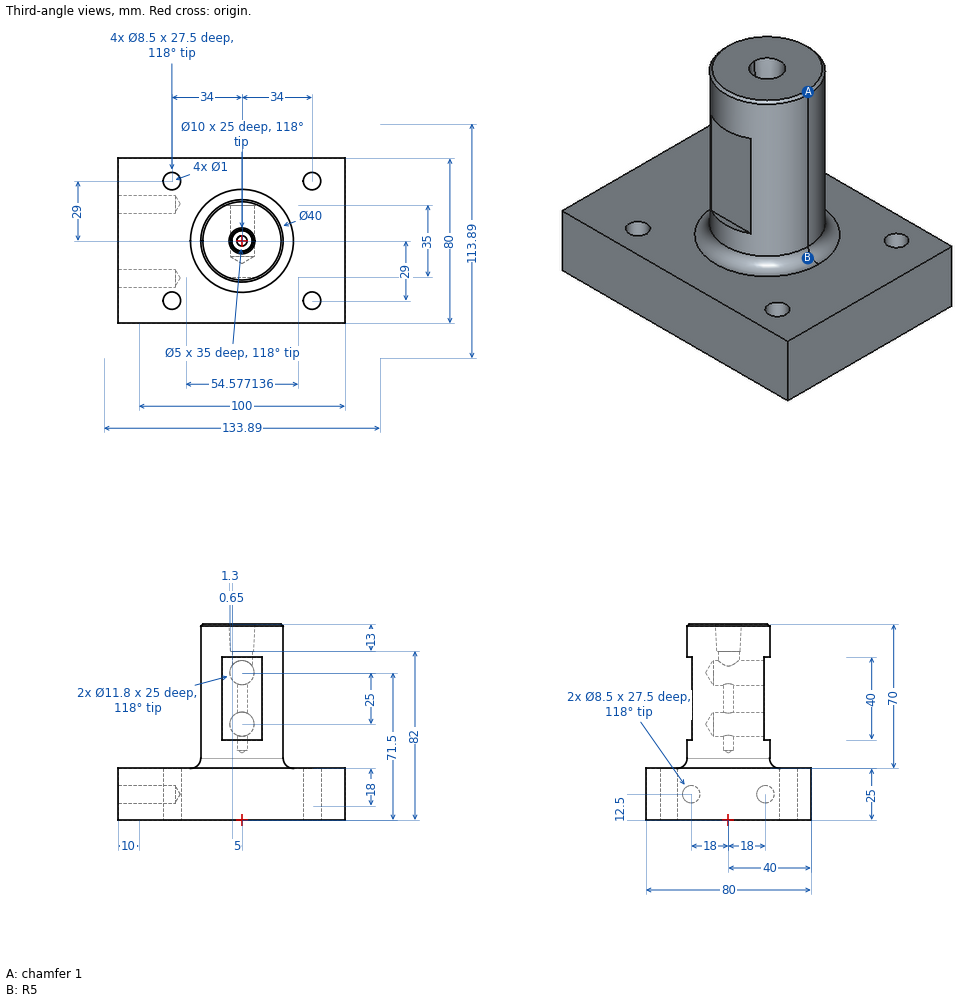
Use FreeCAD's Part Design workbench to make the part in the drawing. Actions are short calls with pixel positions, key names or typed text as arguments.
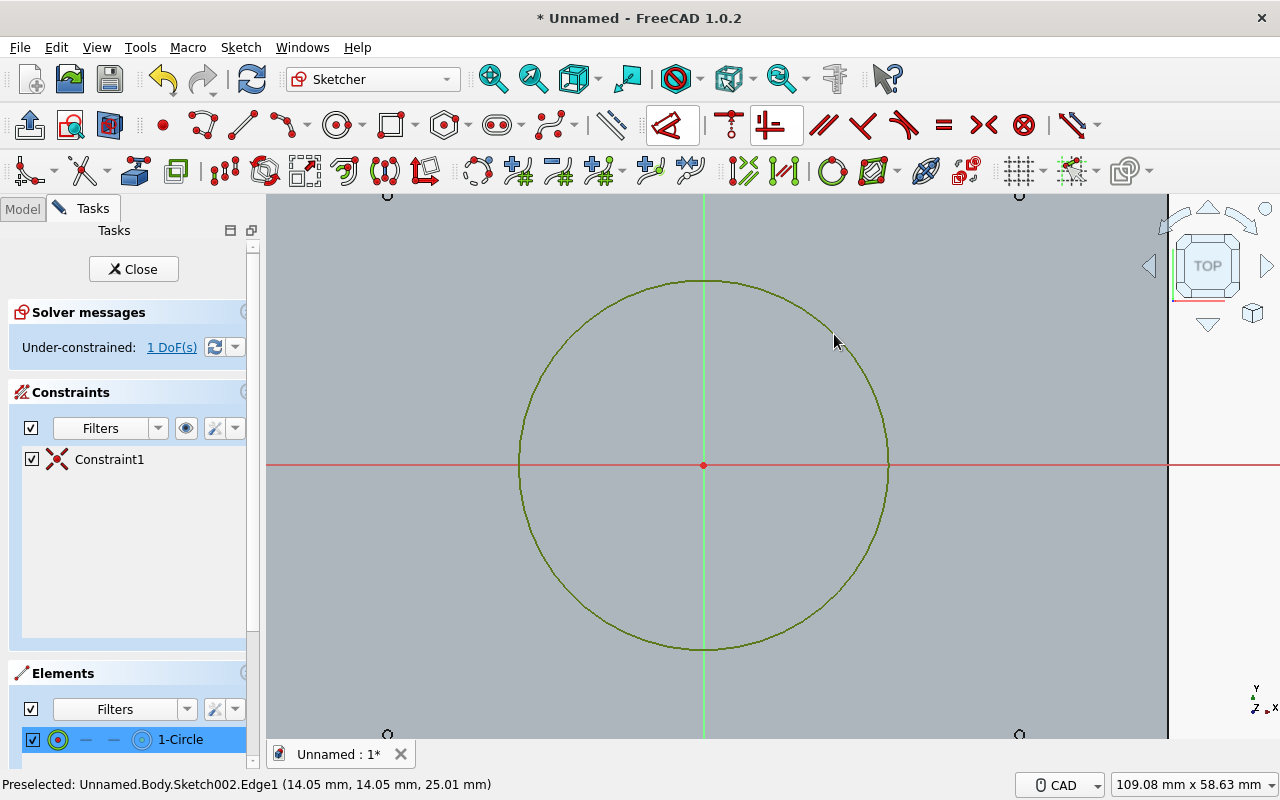
click(694, 126)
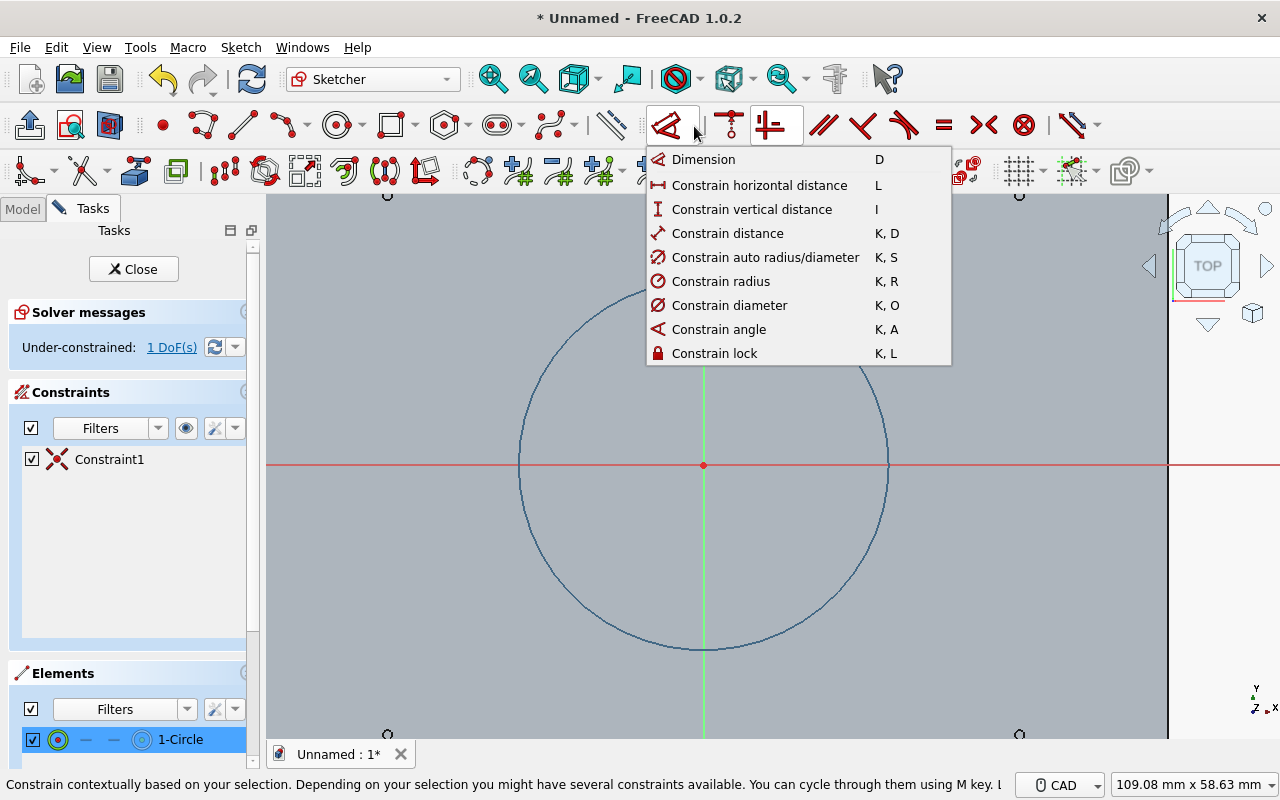
click(799, 305)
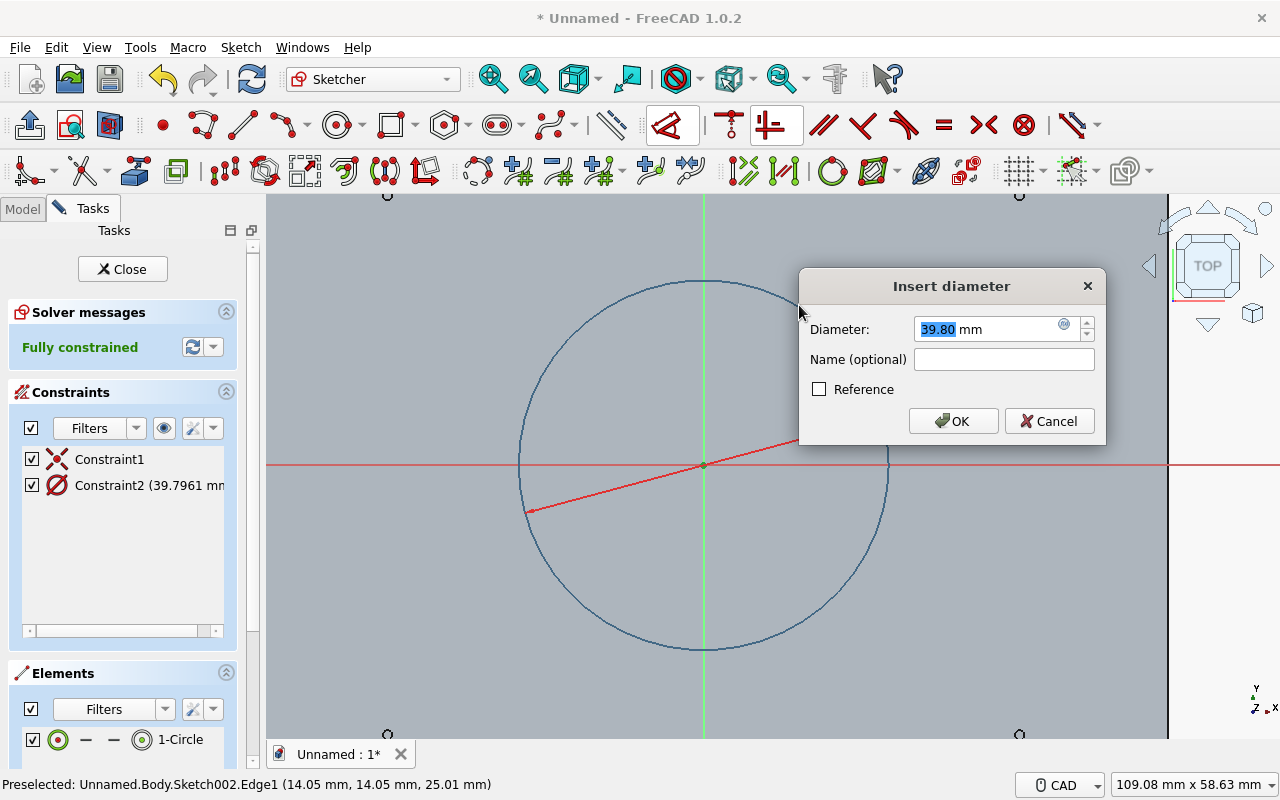
text(40)
key(Return)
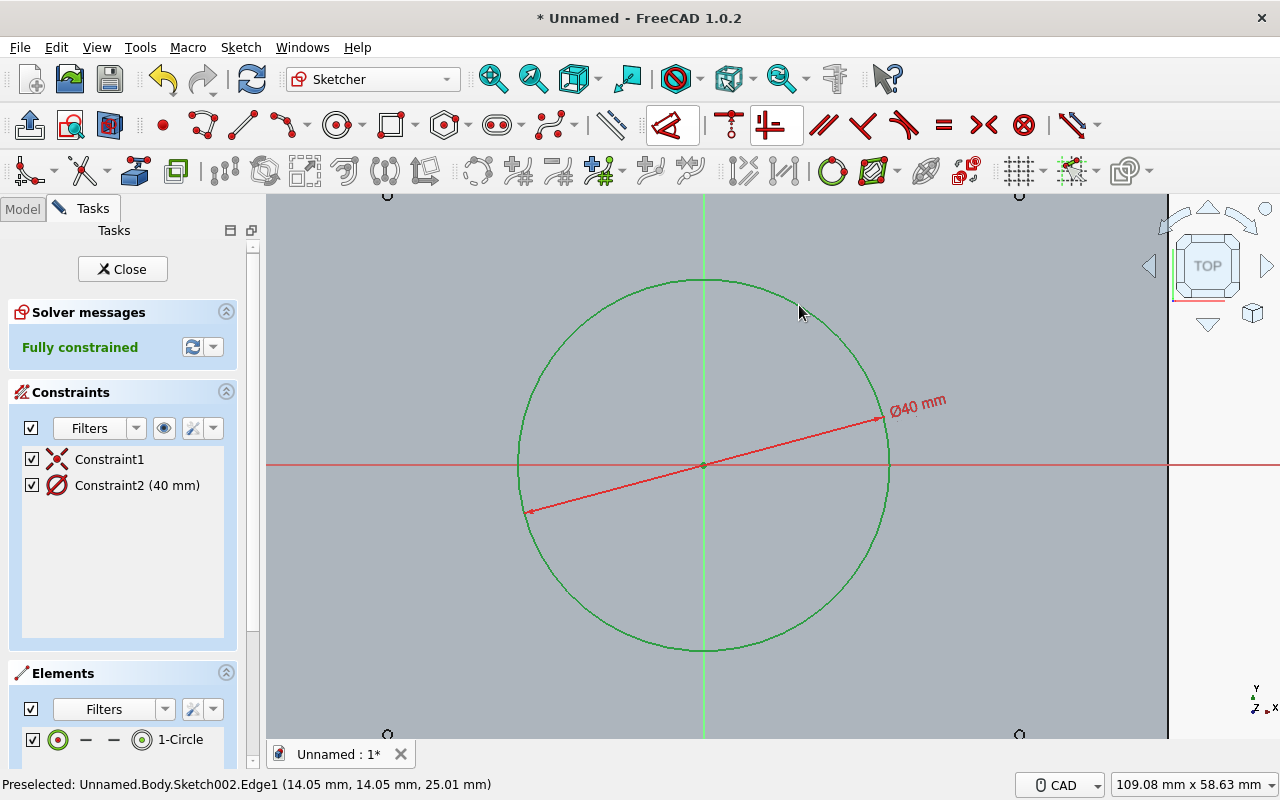
click(123, 269)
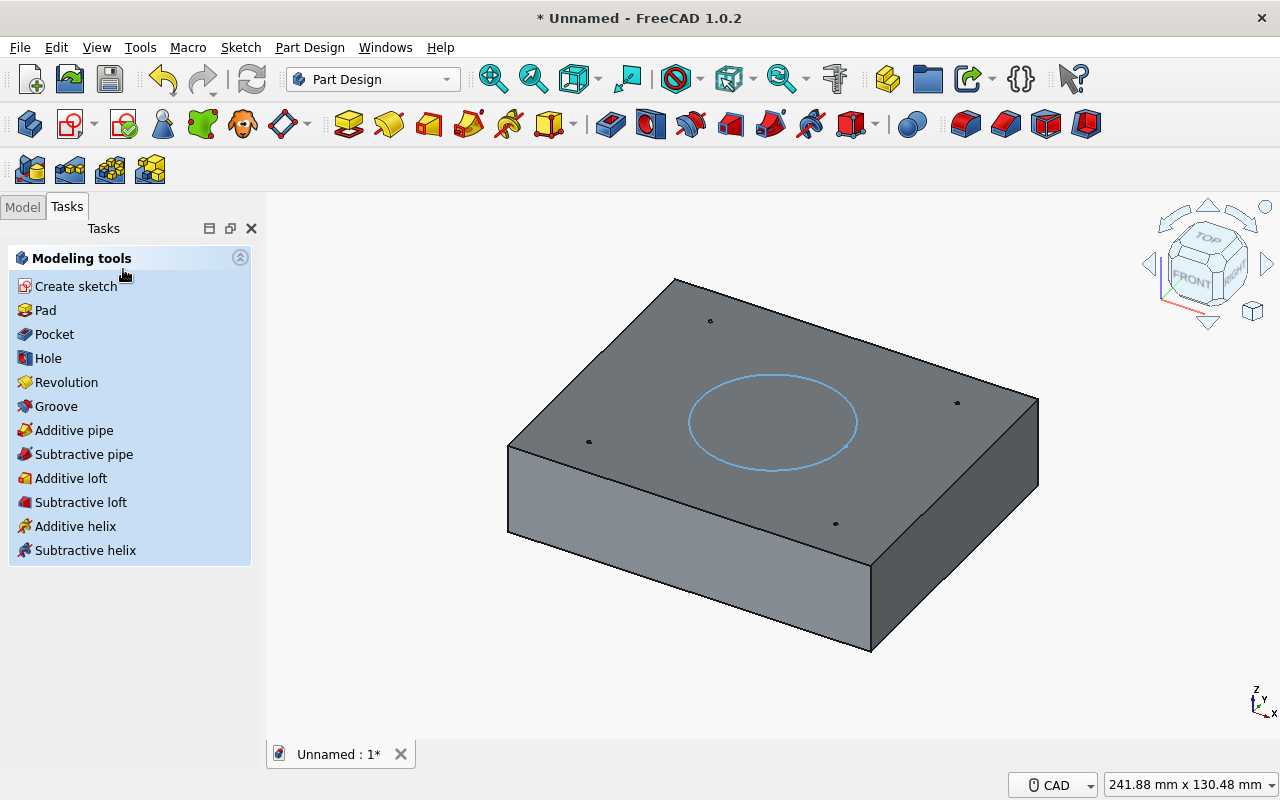
click(350, 124)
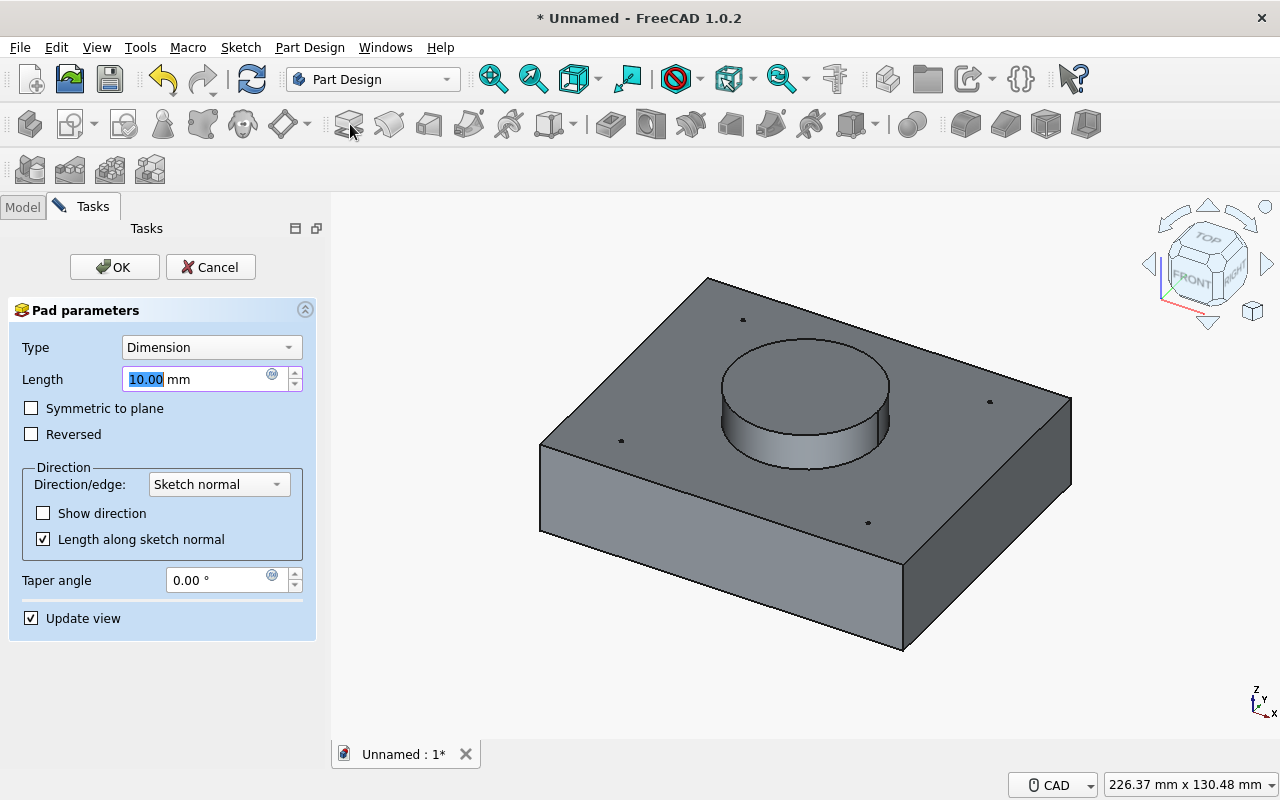
text(70)
key(Tab)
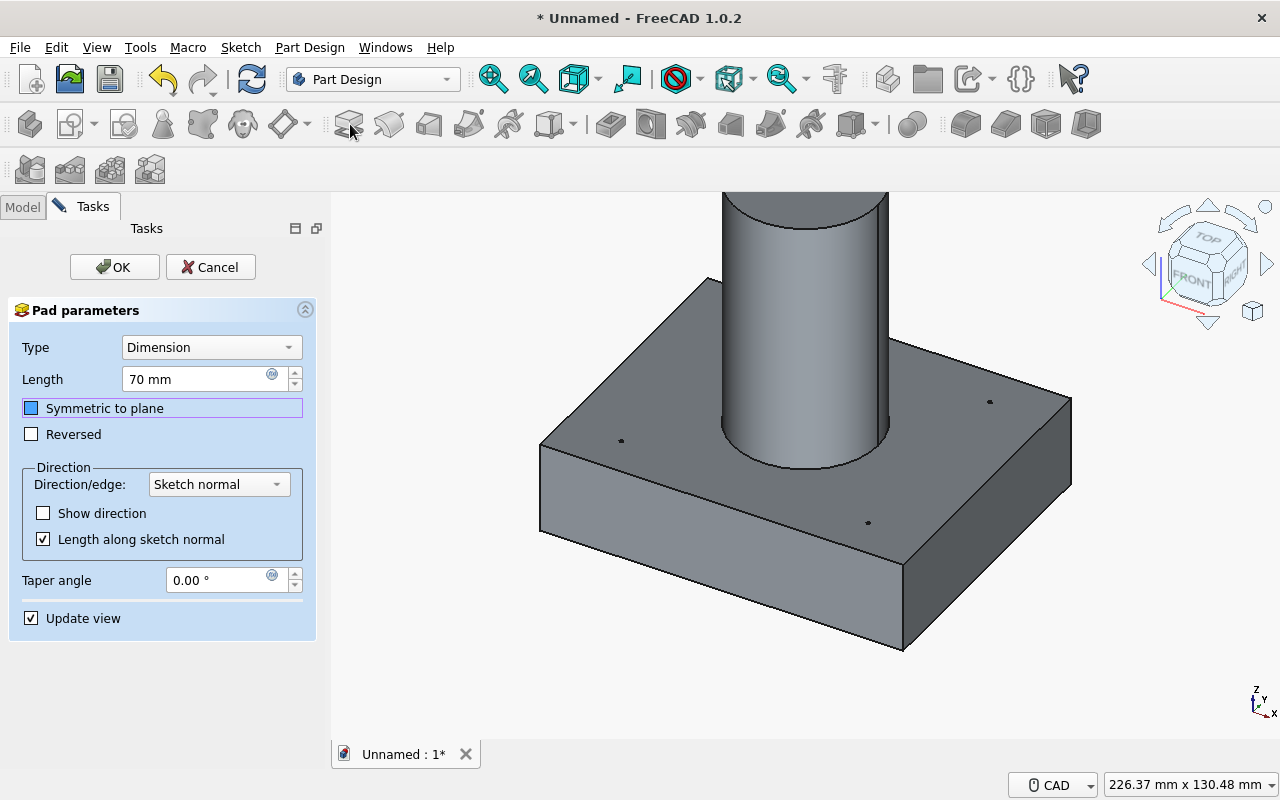
click(115, 267)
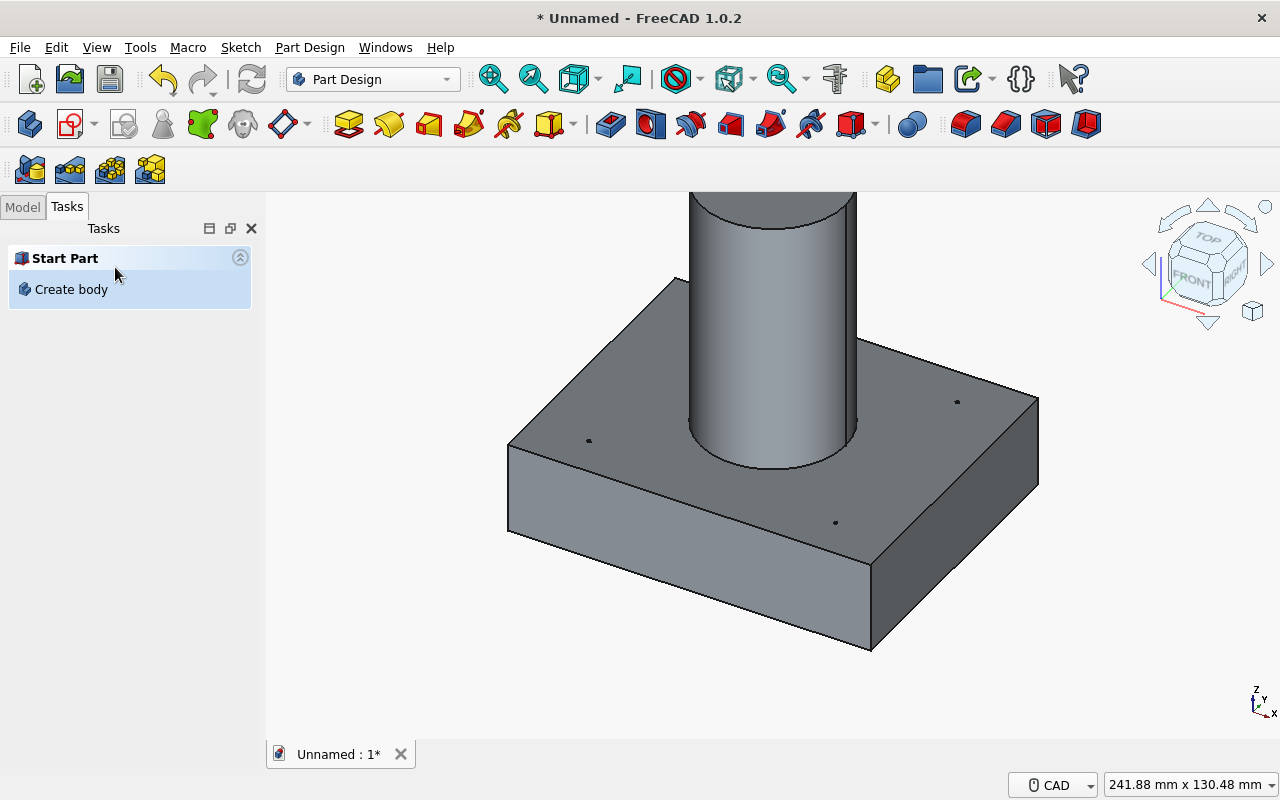
click(494, 80)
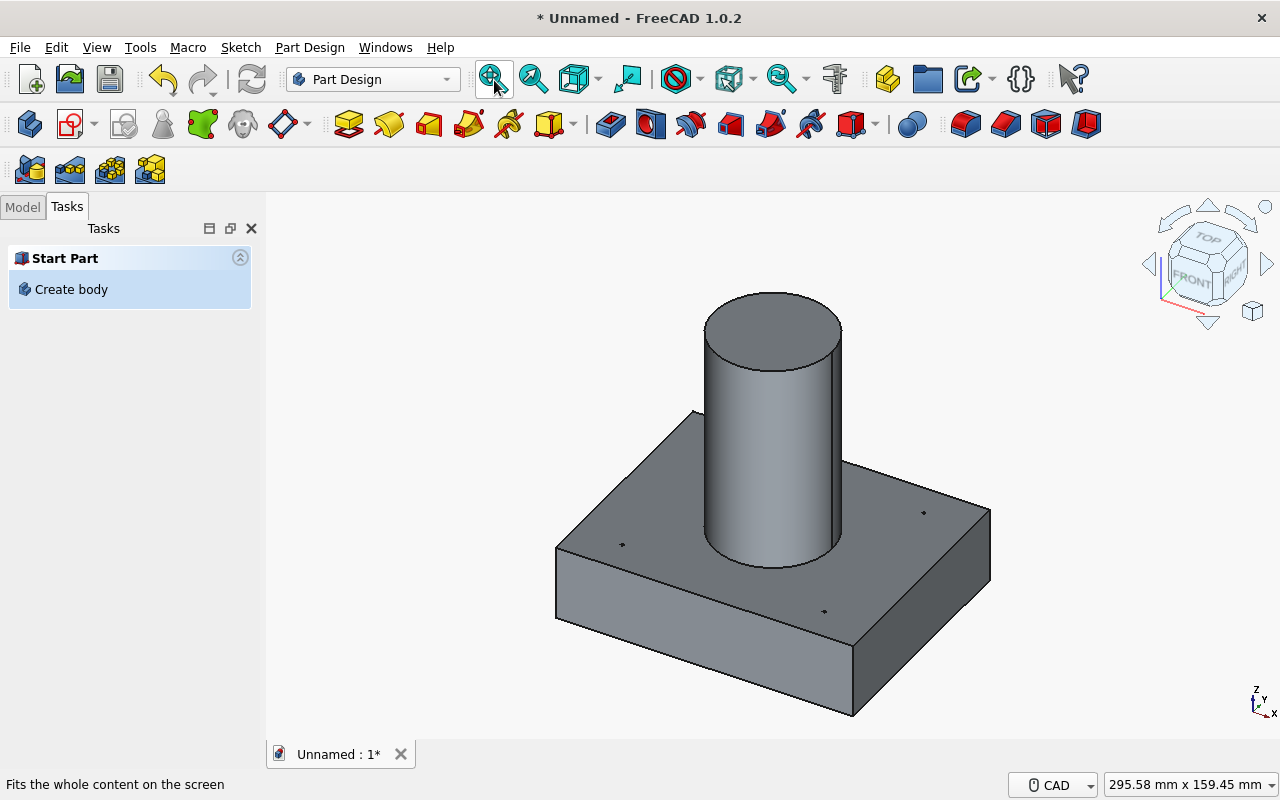
click(773, 331)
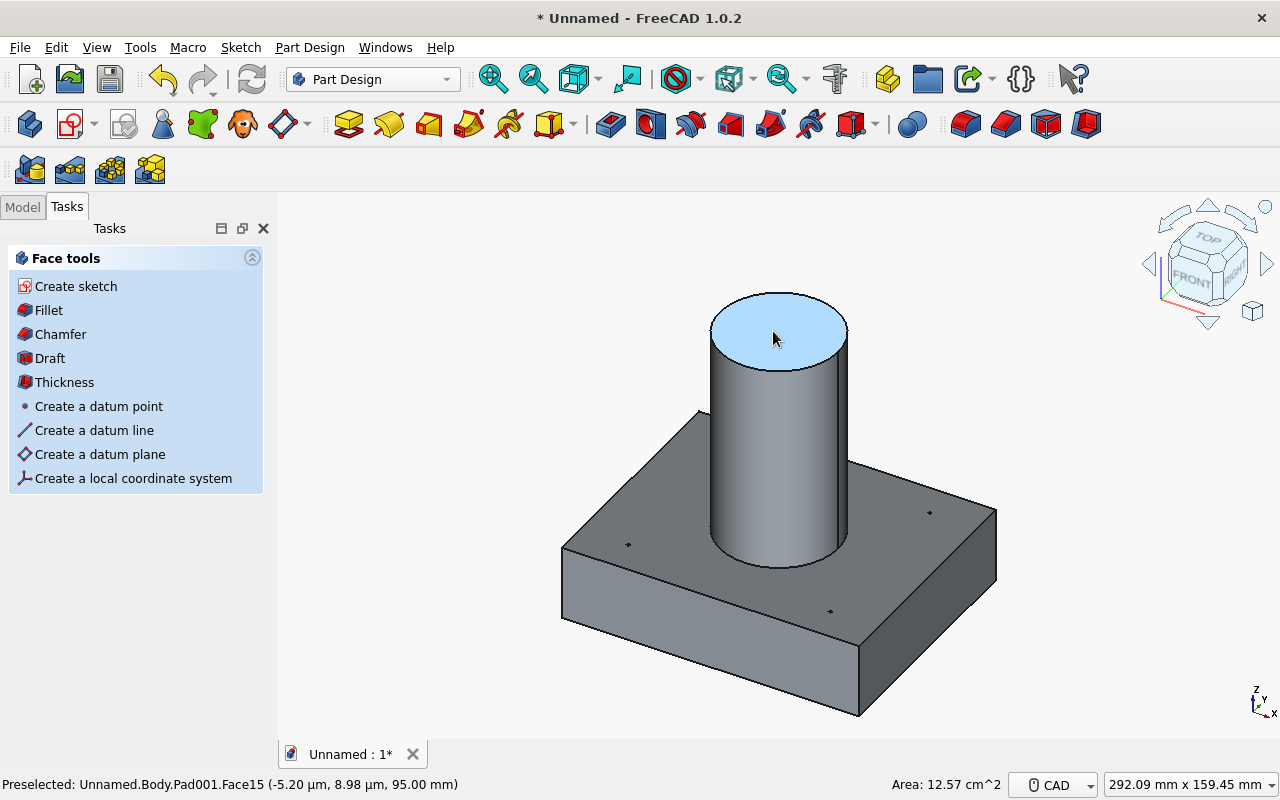
click(70, 124)